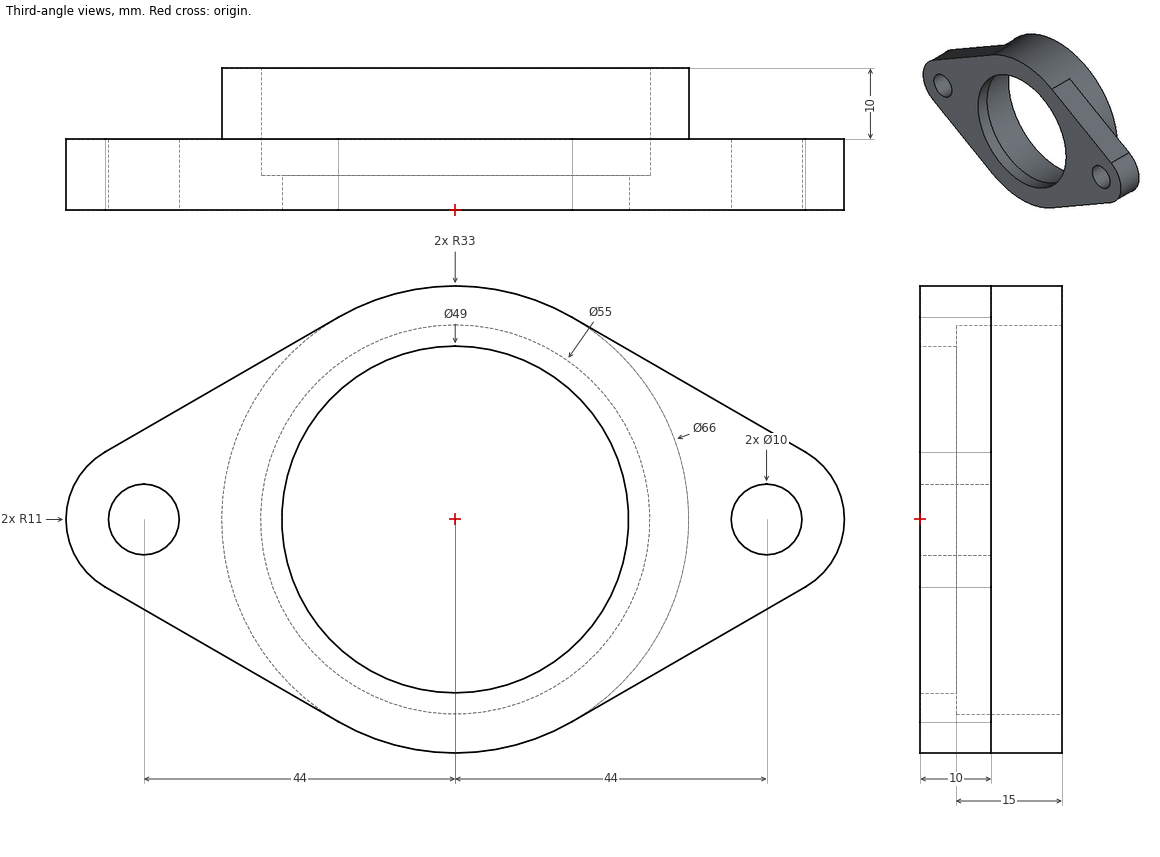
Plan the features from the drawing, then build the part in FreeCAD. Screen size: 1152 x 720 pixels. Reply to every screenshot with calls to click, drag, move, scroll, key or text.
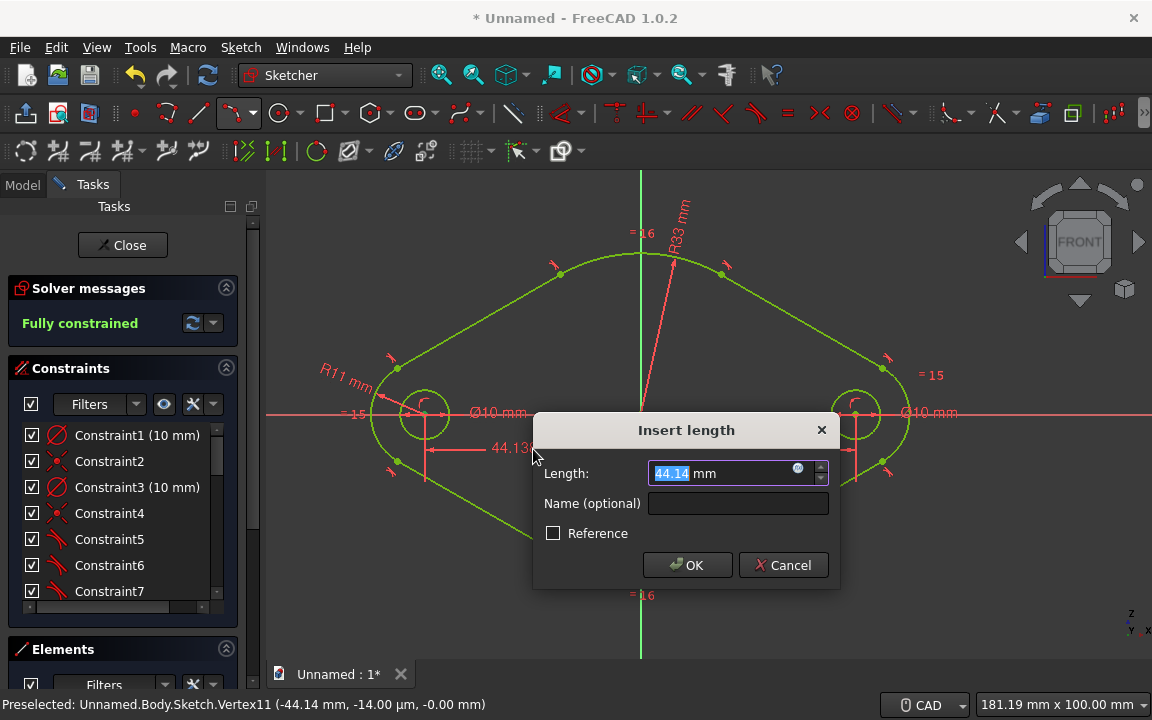
text(44)
key(Return)
key(Escape)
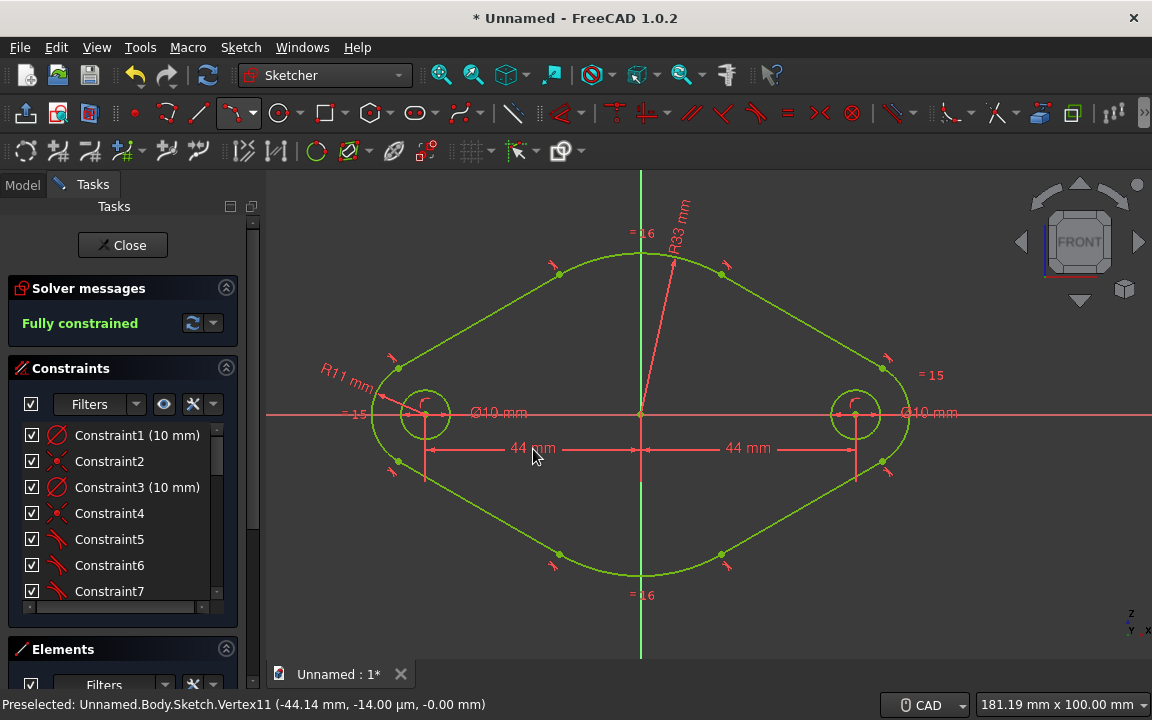
click(123, 245)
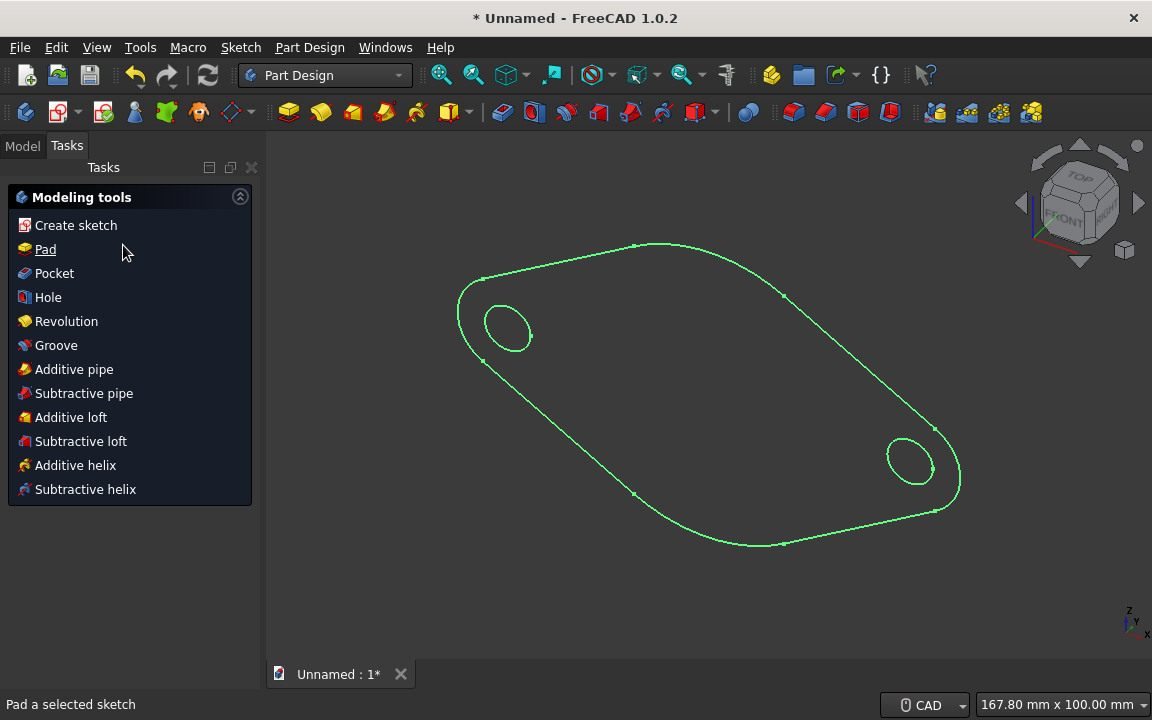
click(290, 112)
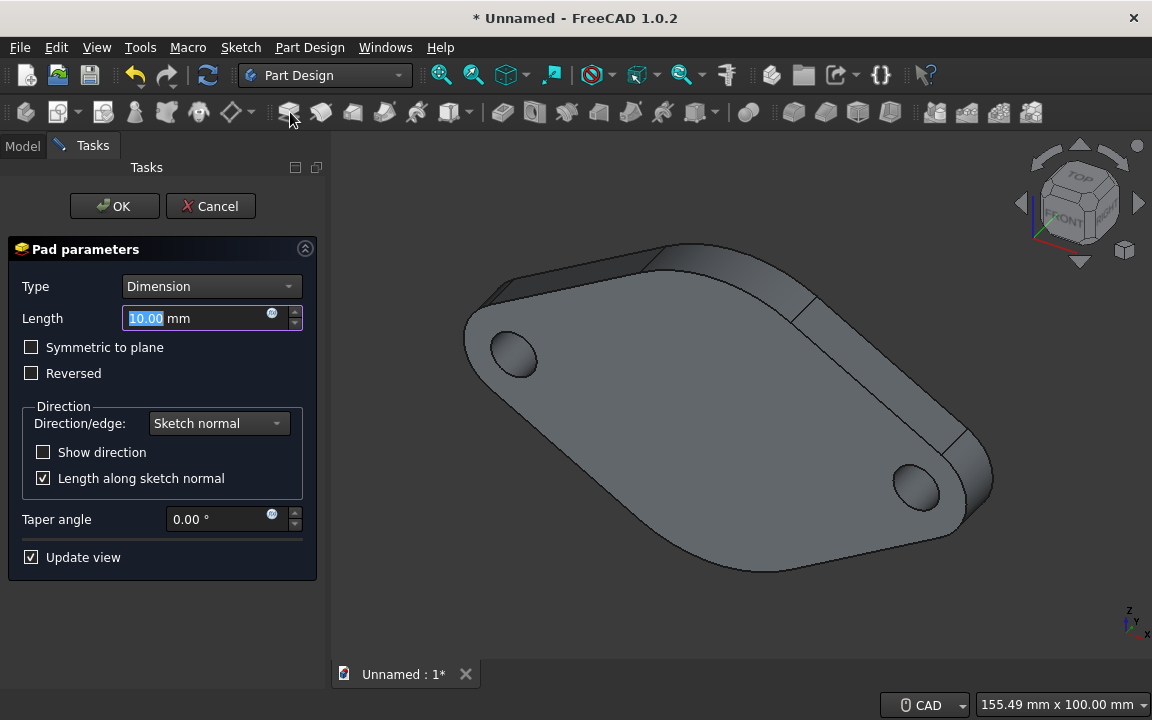
text(10)
key(Tab)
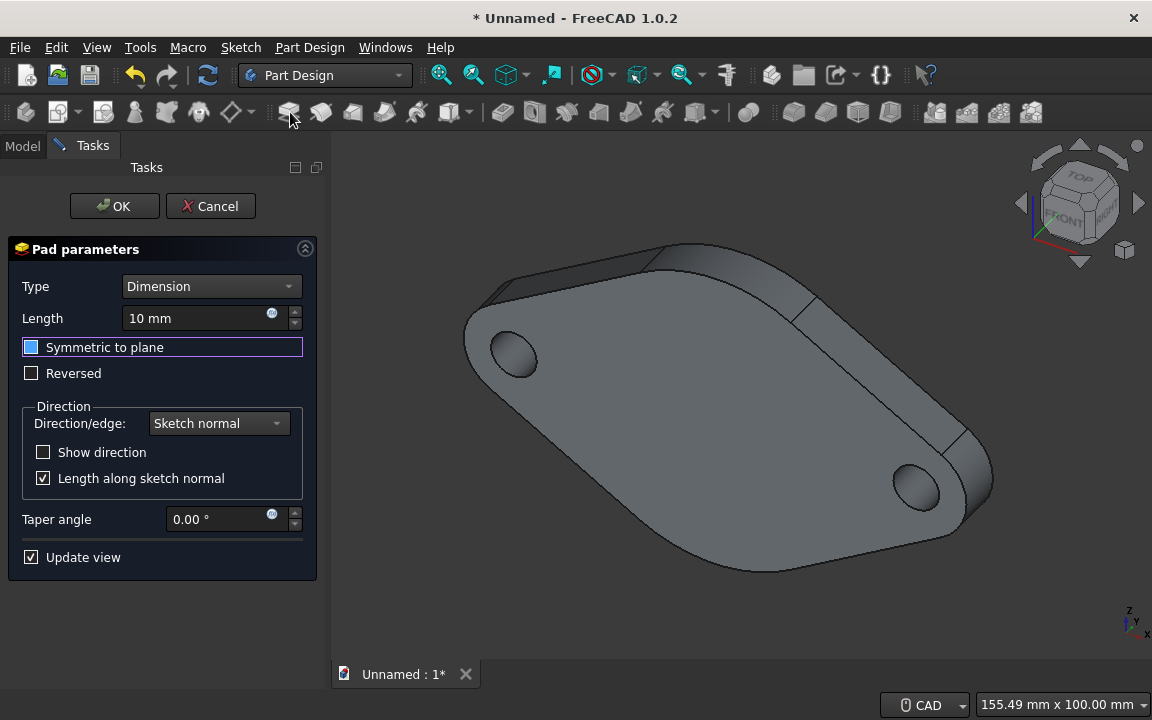
click(30, 373)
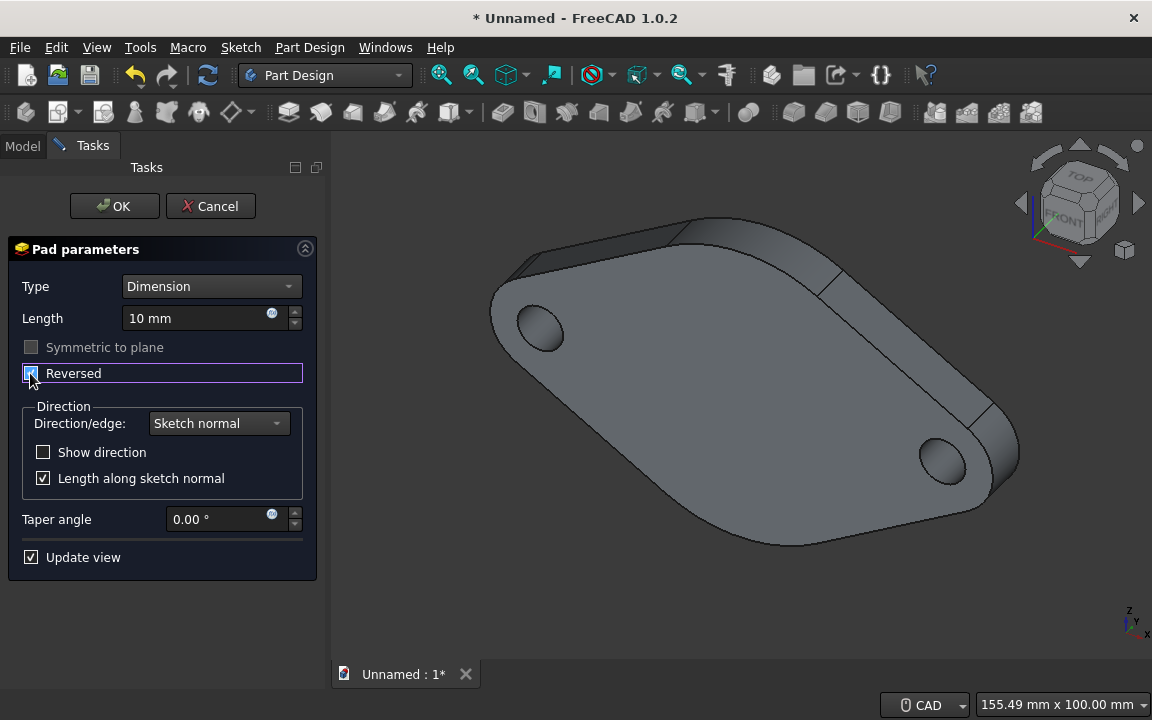
click(115, 206)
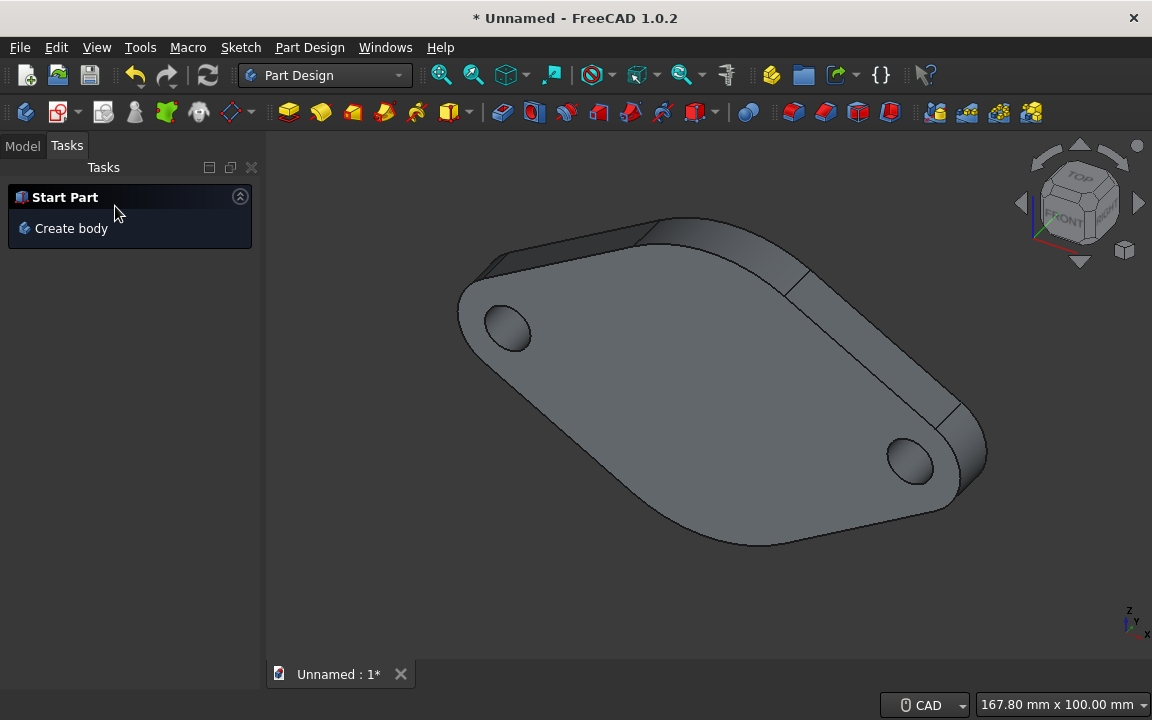
key(4)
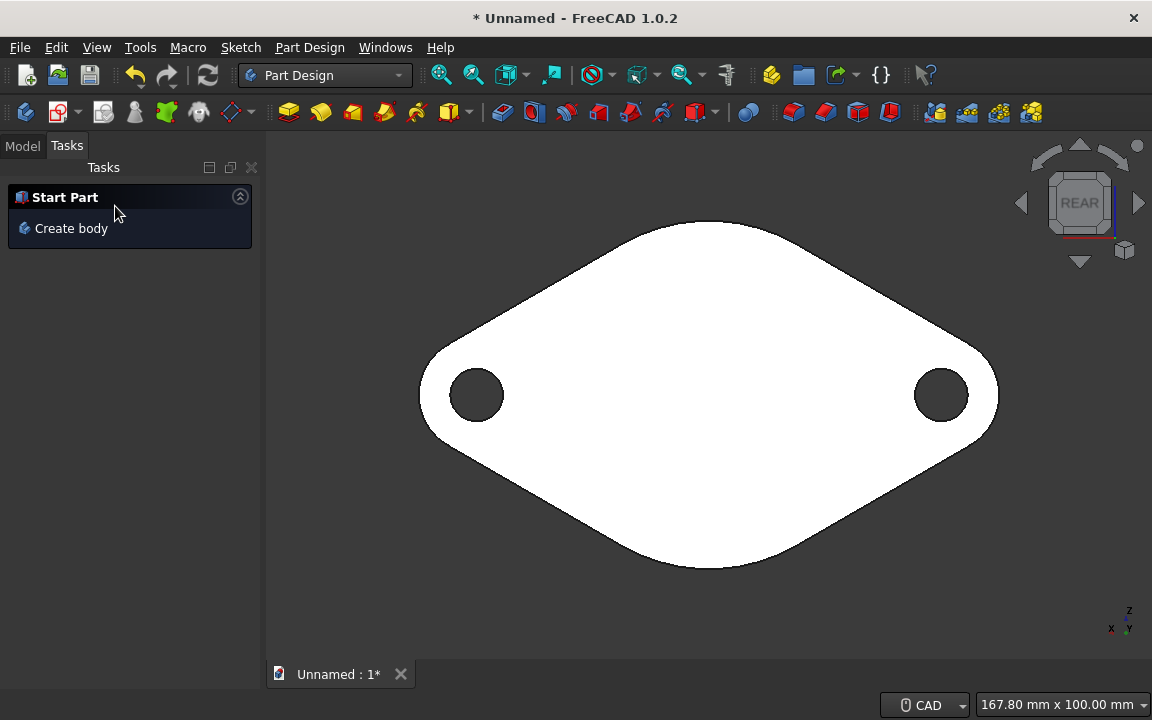
click(709, 394)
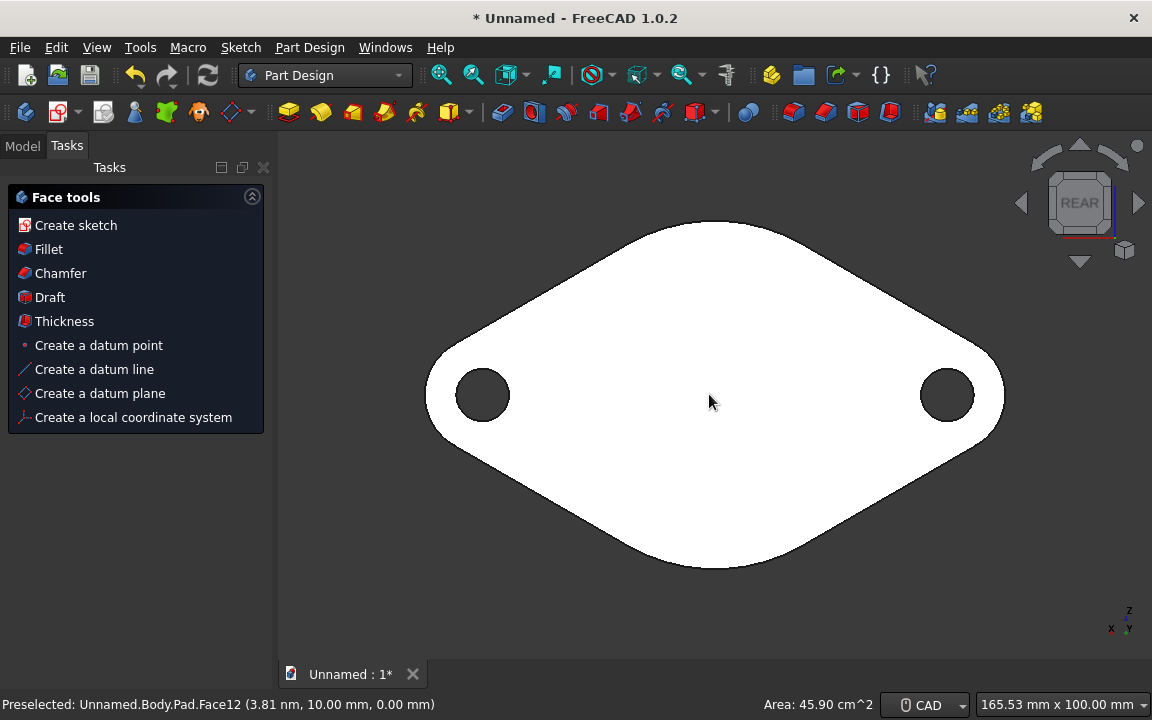
click(58, 112)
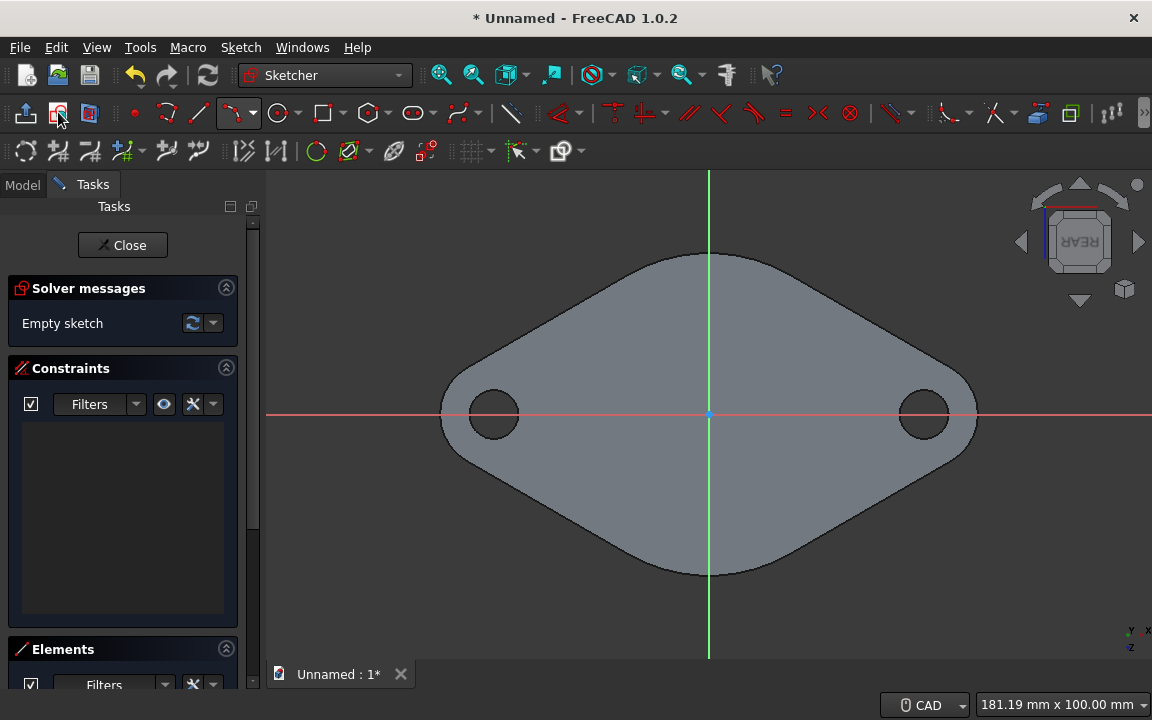
click(278, 114)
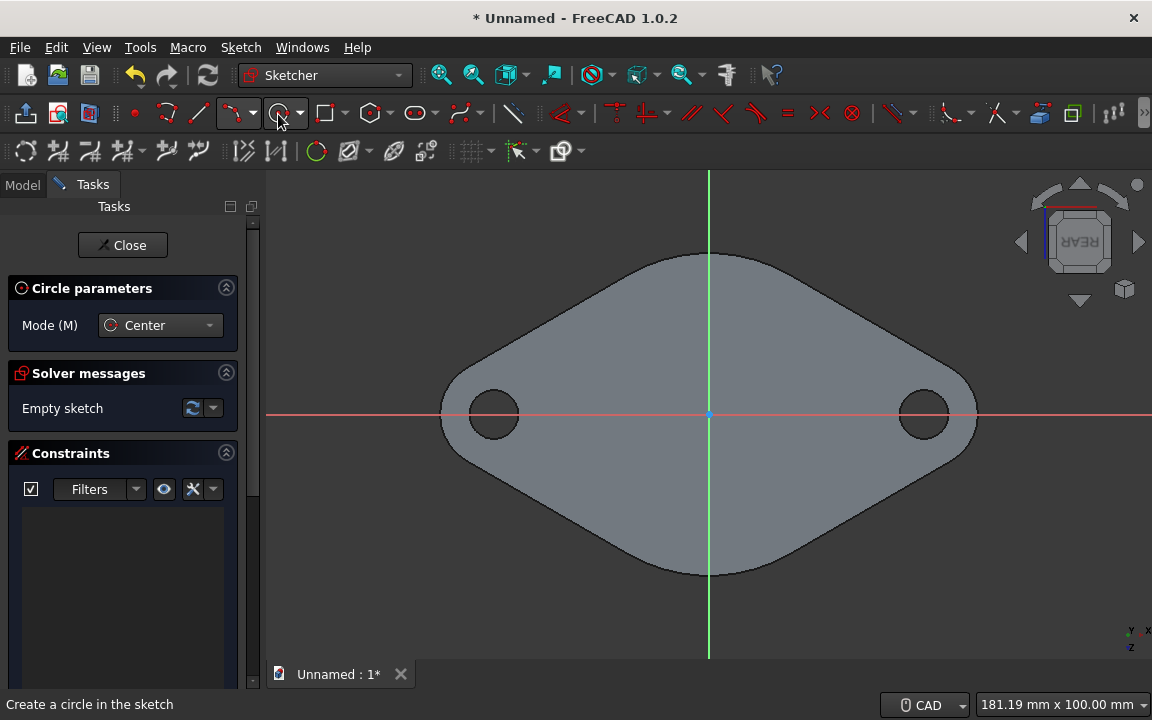
click(709, 415)
move(823, 300)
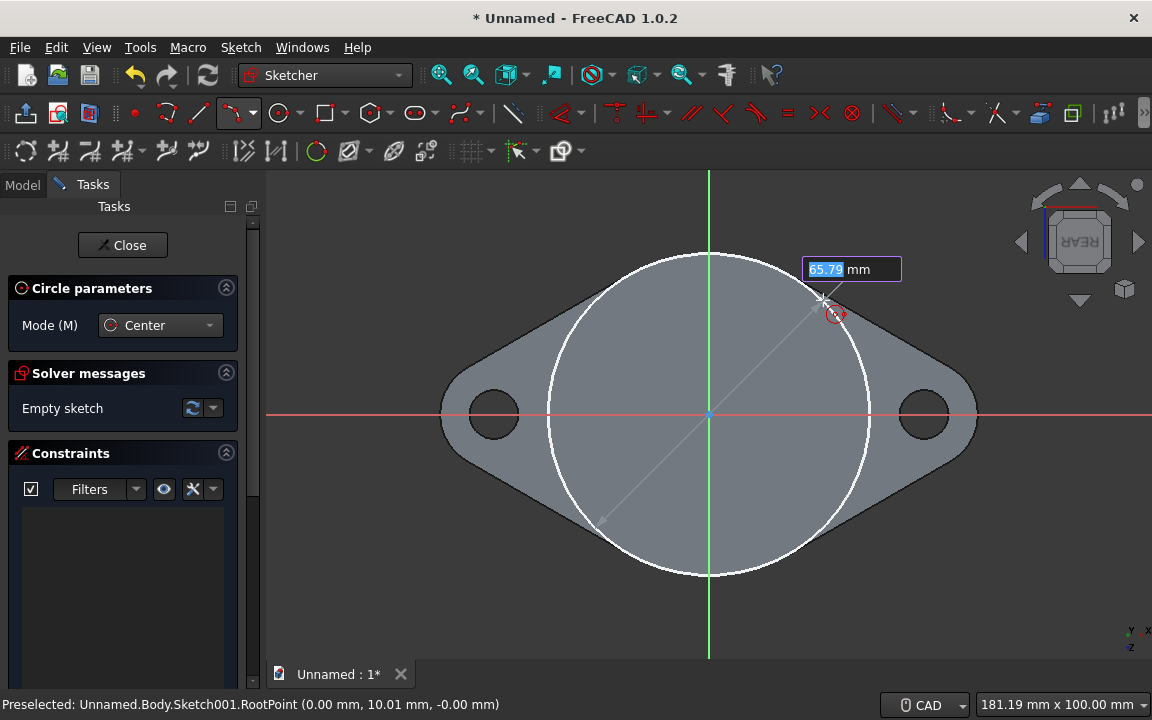
text(66)
key(Return)
key(Escape)